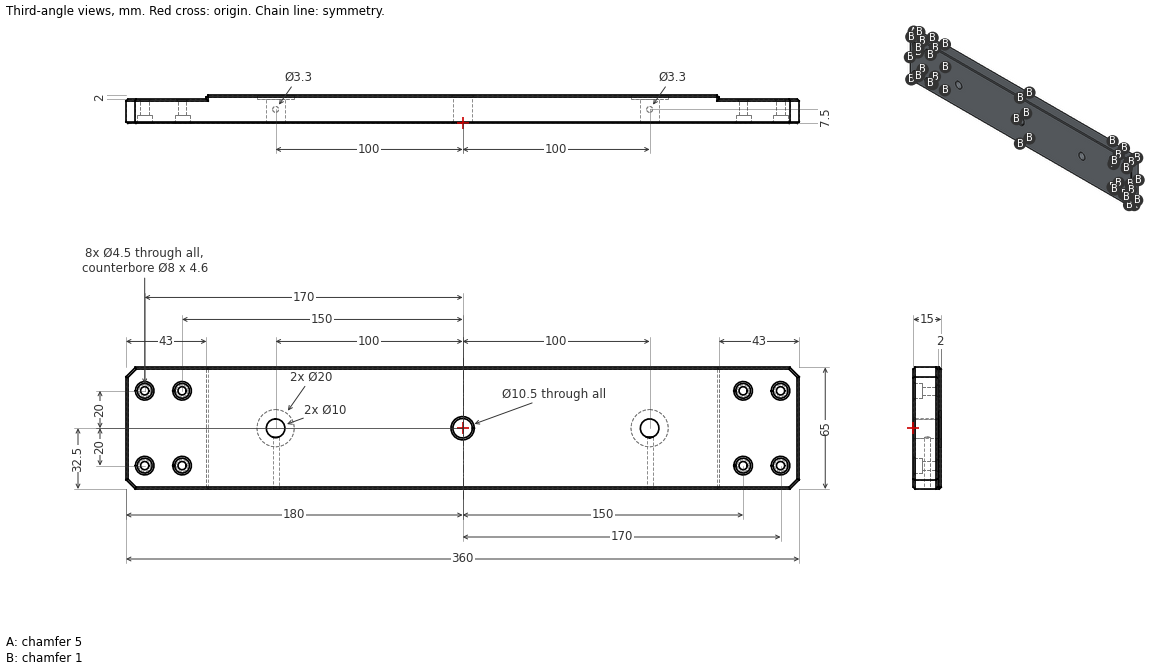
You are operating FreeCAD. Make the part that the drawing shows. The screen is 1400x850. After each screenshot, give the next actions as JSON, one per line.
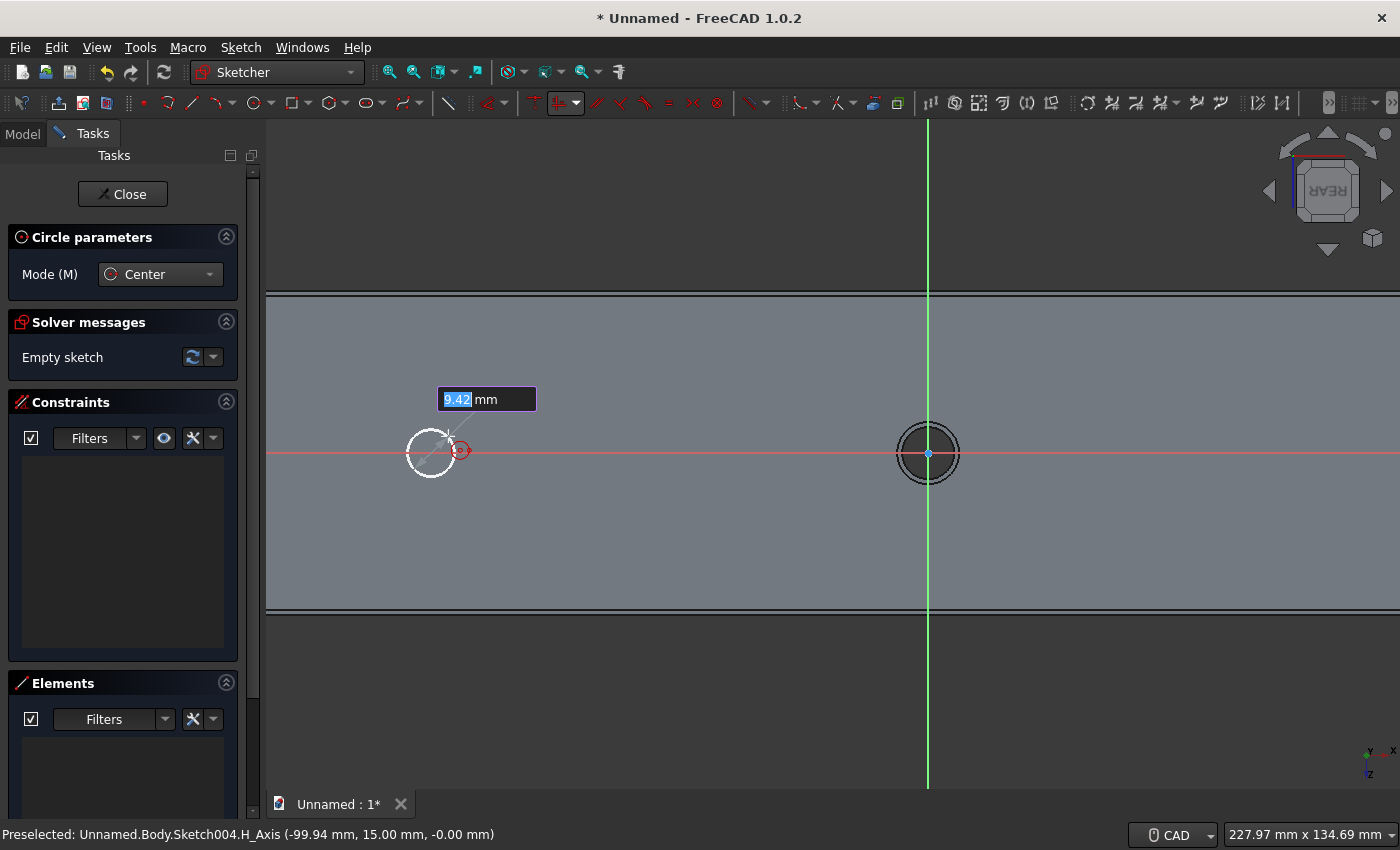
{"action": "type", "text": "10"}
{"action": "key", "text": "Return"}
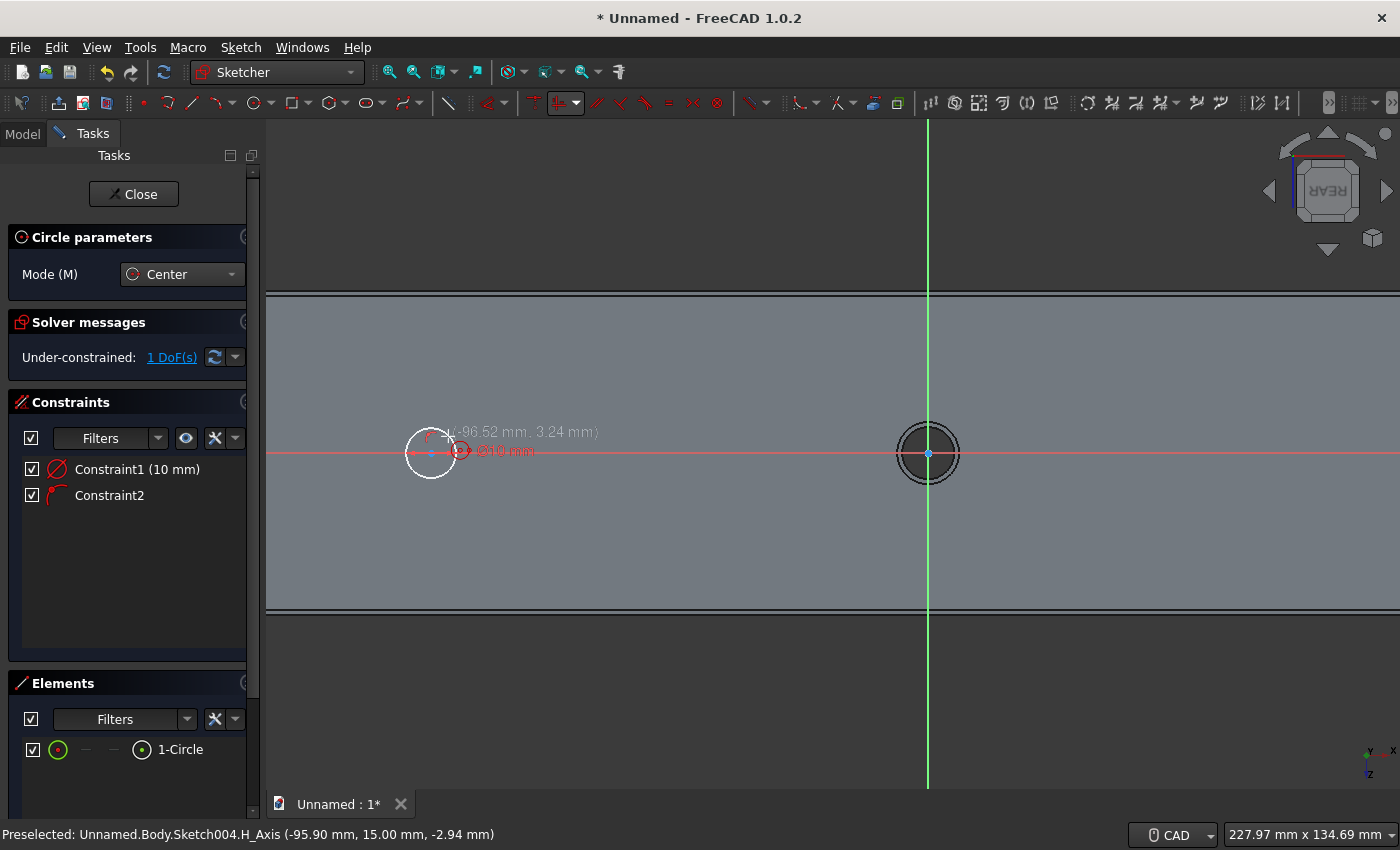
{"action": "scroll", "coordinate": [432, 456], "scroll_direction": "down", "scroll_amount": 2}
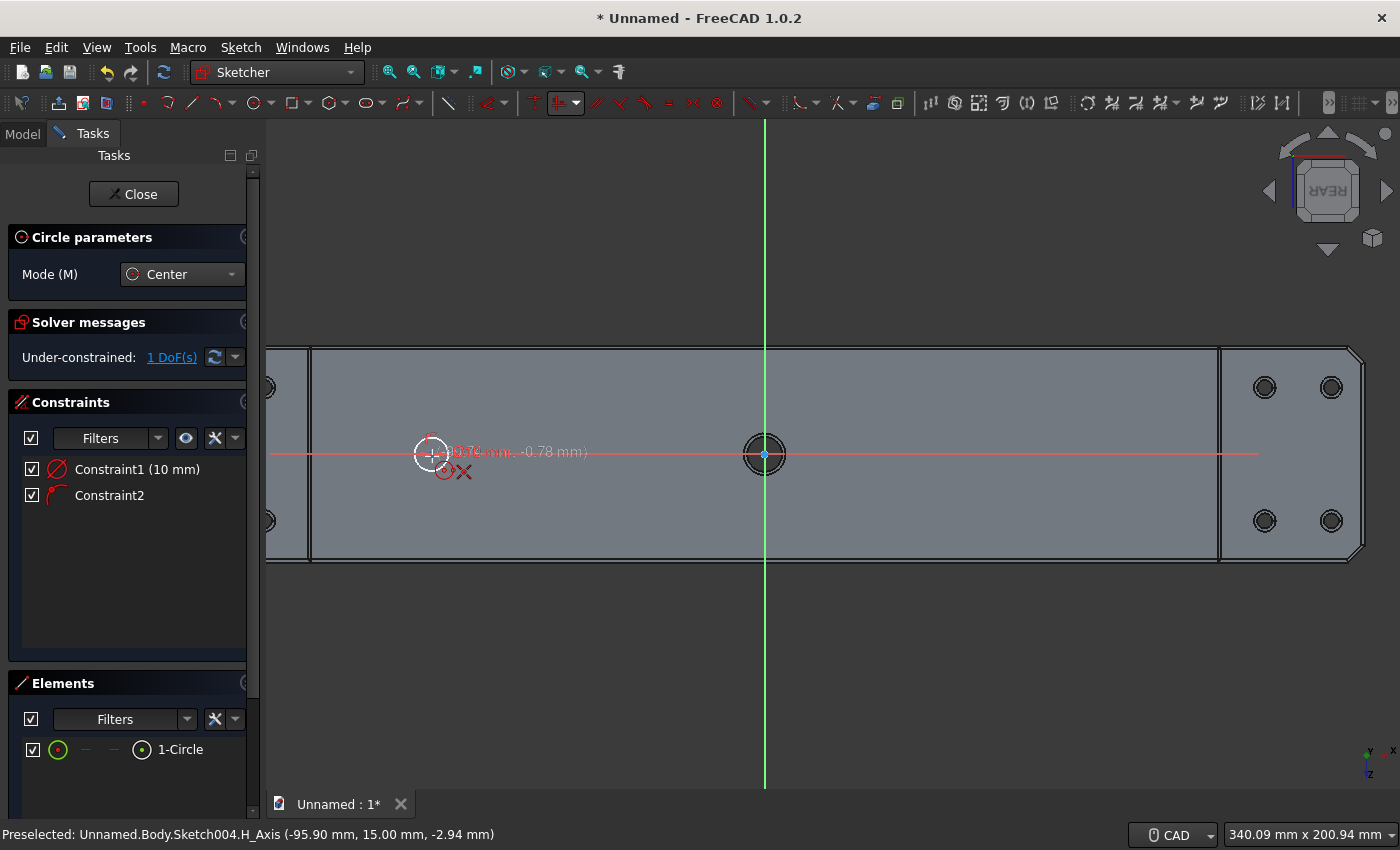
{"action": "scroll", "coordinate": [1098, 454], "scroll_direction": "up", "scroll_amount": 2}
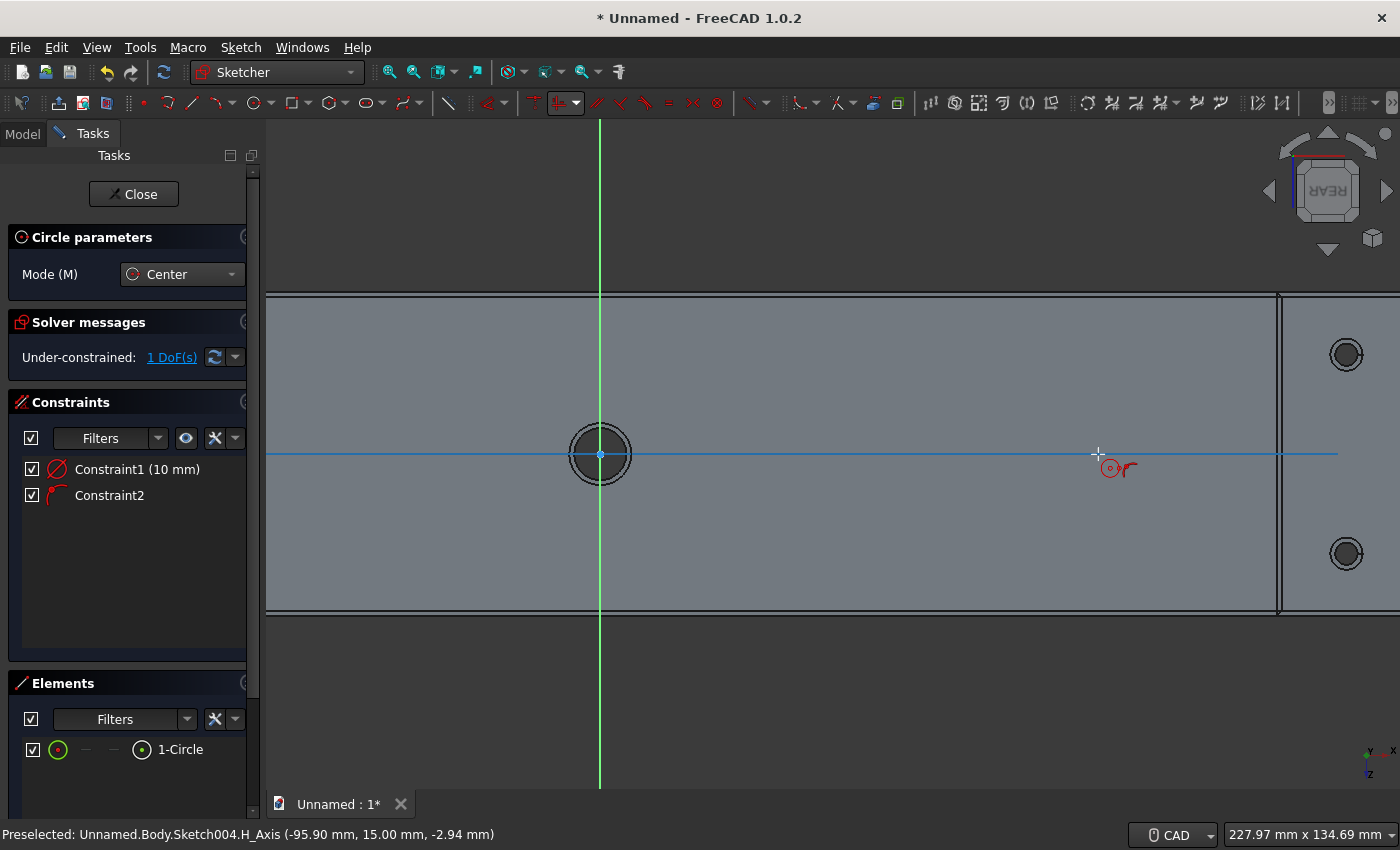
{"action": "left_click", "coordinate": [1098, 454]}
{"action": "mouse_move", "coordinate": [1115, 437]}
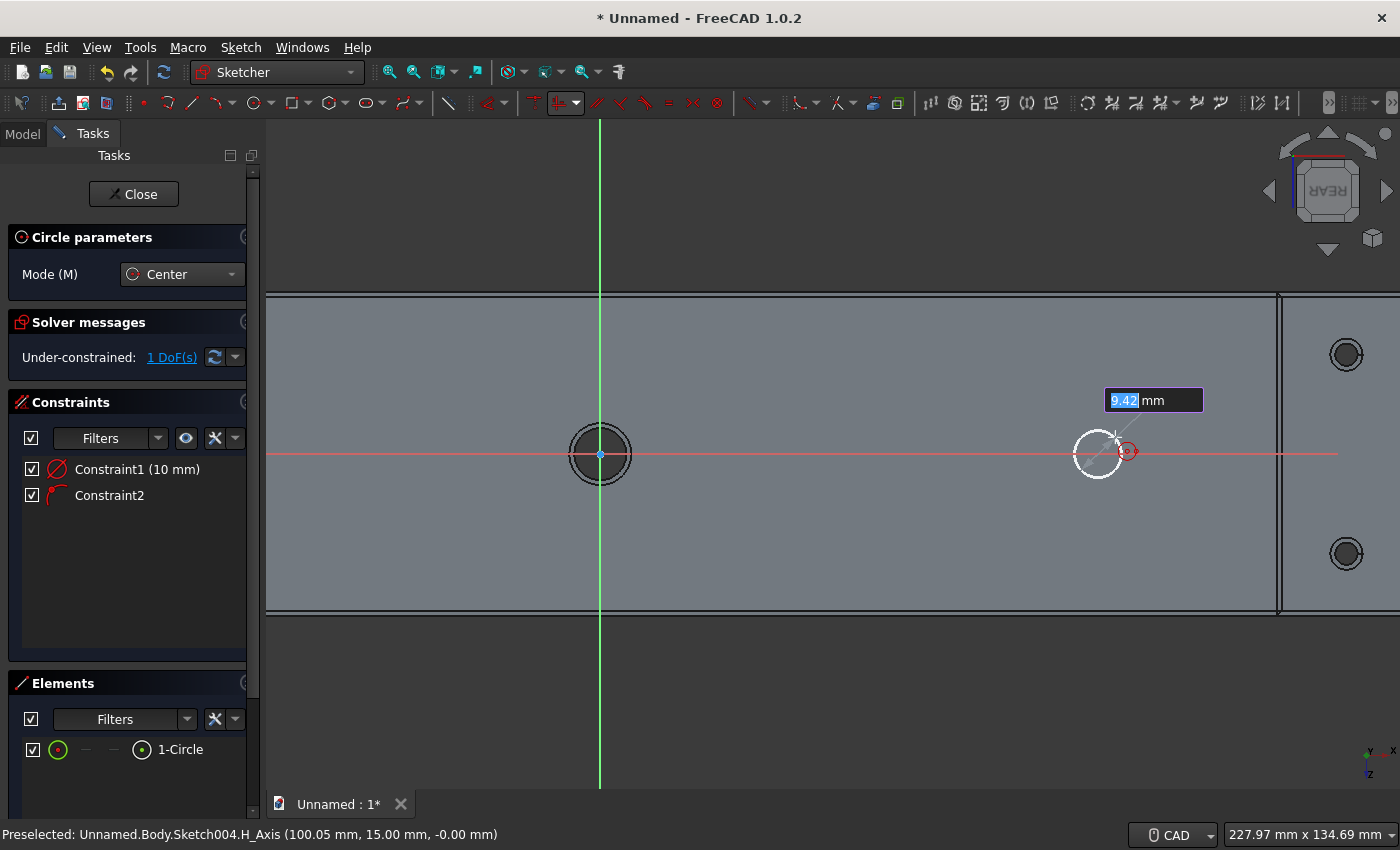
{"action": "type", "text": "10"}
{"action": "key", "text": "Return"}
{"action": "key", "text": "Escape"}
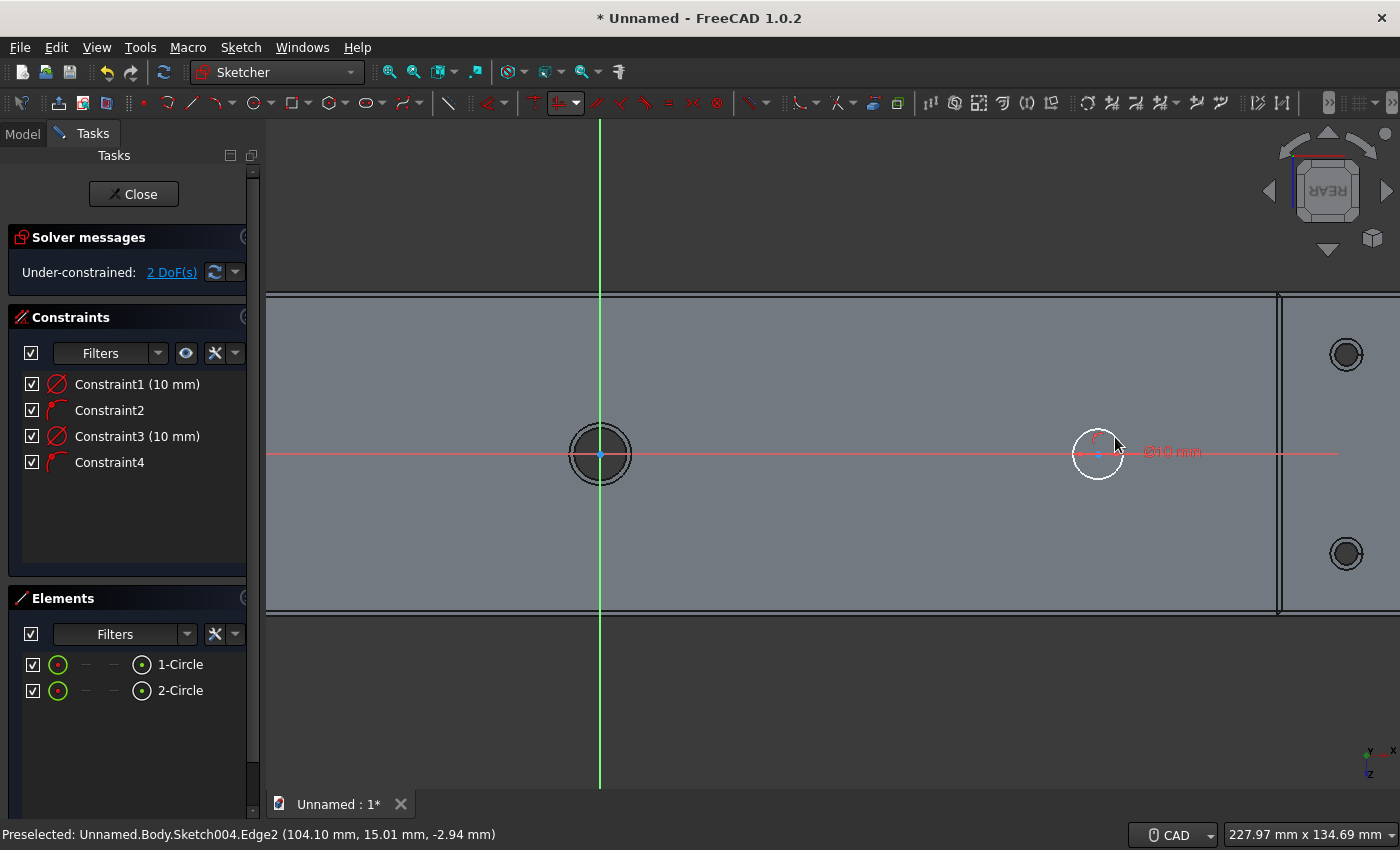
{"action": "left_click", "coordinate": [488, 104]}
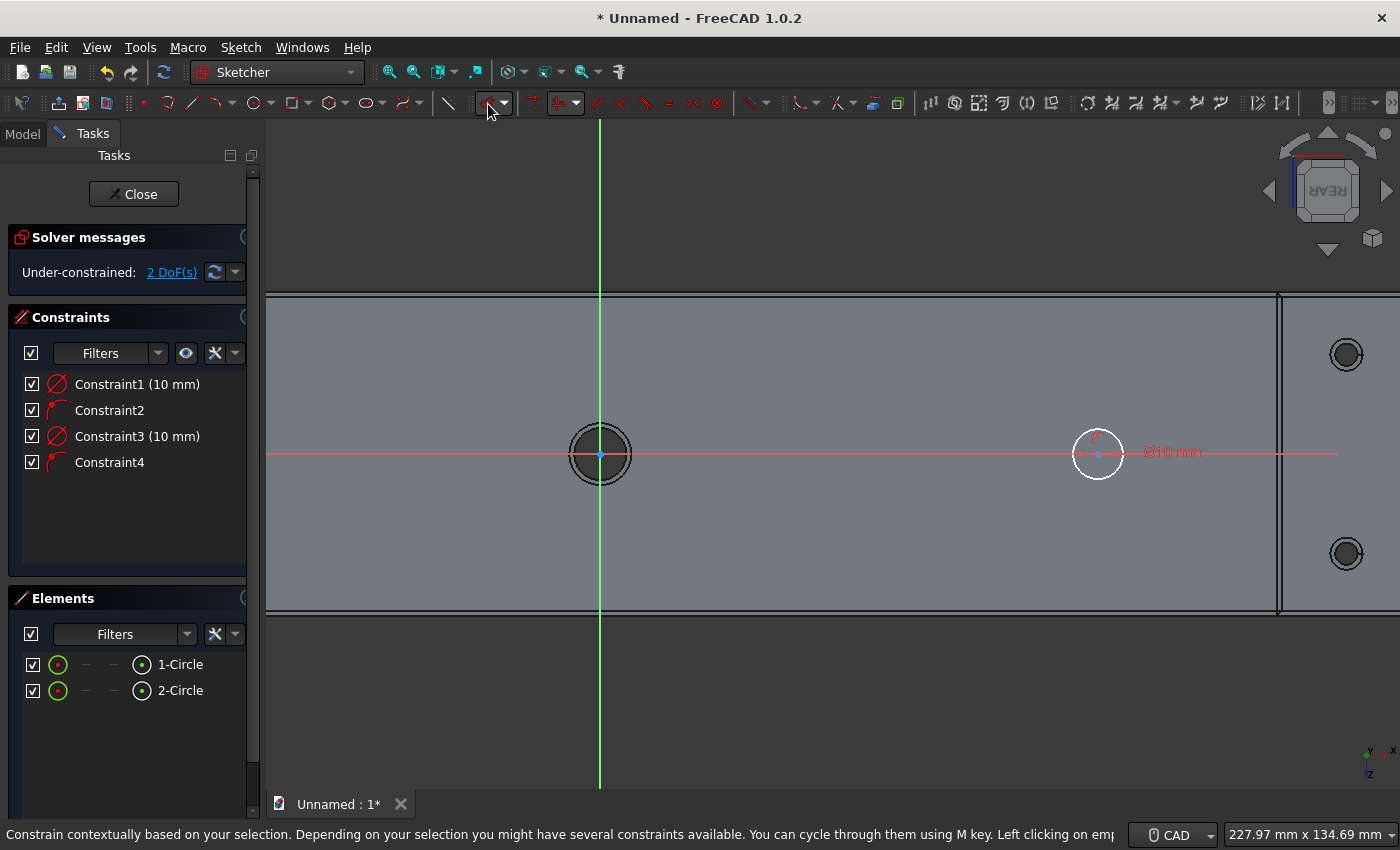
{"action": "scroll", "coordinate": [1098, 454], "scroll_direction": "down", "scroll_amount": 2}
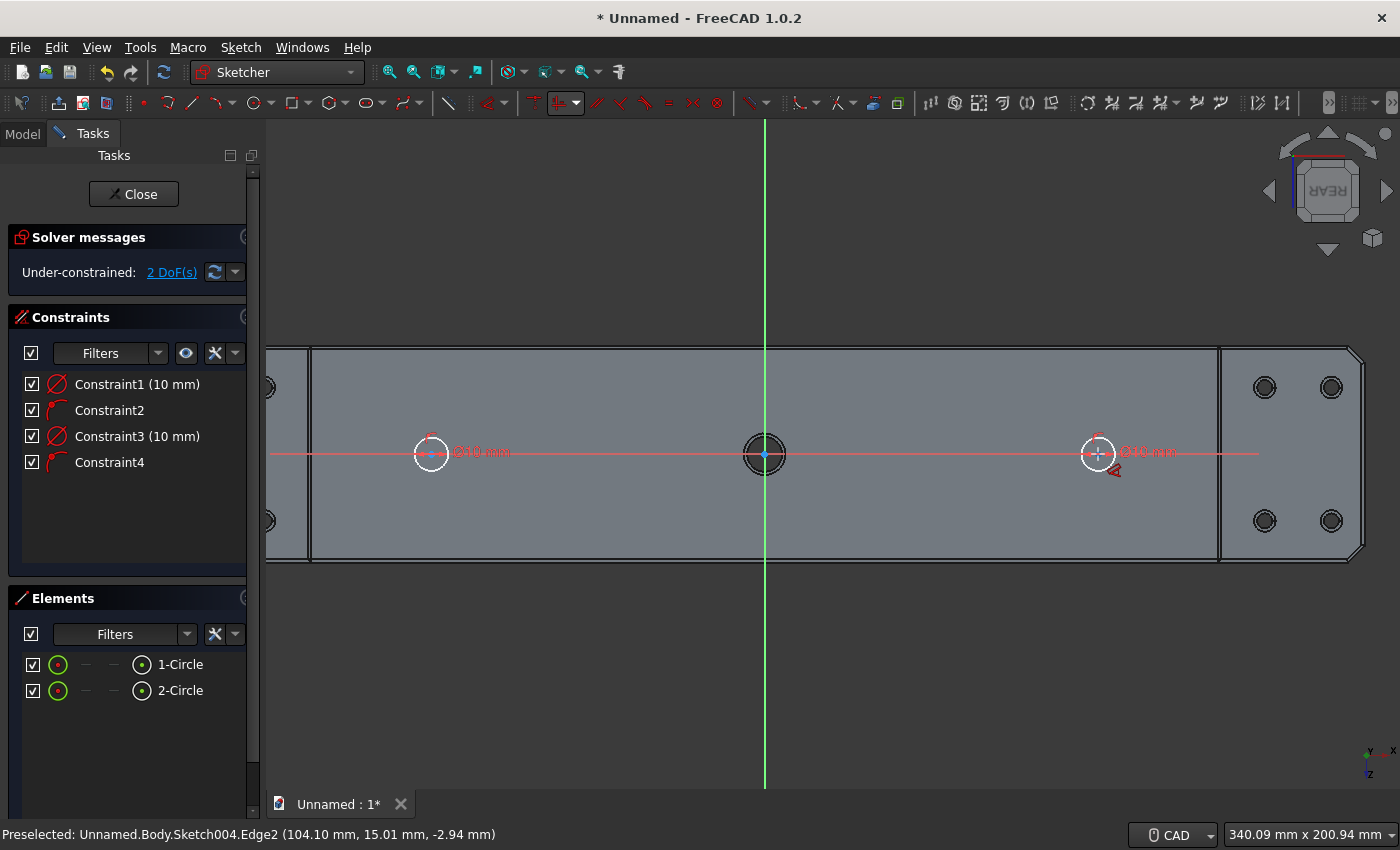
{"action": "left_click", "coordinate": [431, 454]}
{"action": "left_click", "coordinate": [598, 488]}